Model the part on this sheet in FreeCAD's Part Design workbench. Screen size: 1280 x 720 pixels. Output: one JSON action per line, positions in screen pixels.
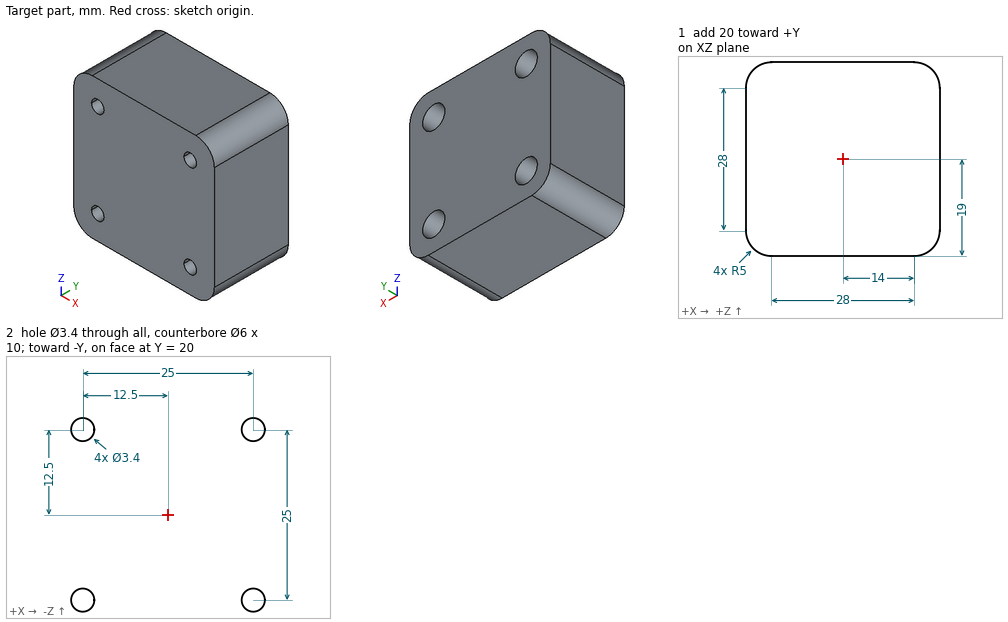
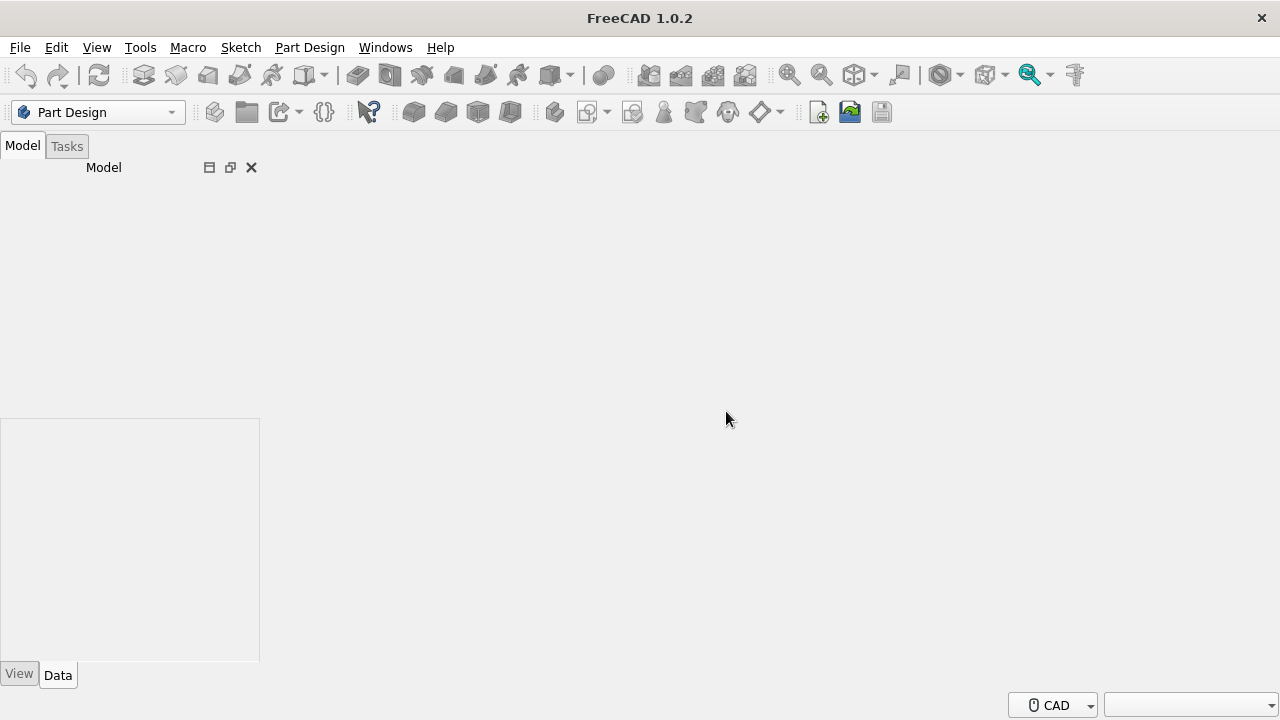
{"action": "left_click", "coordinate": [818, 112]}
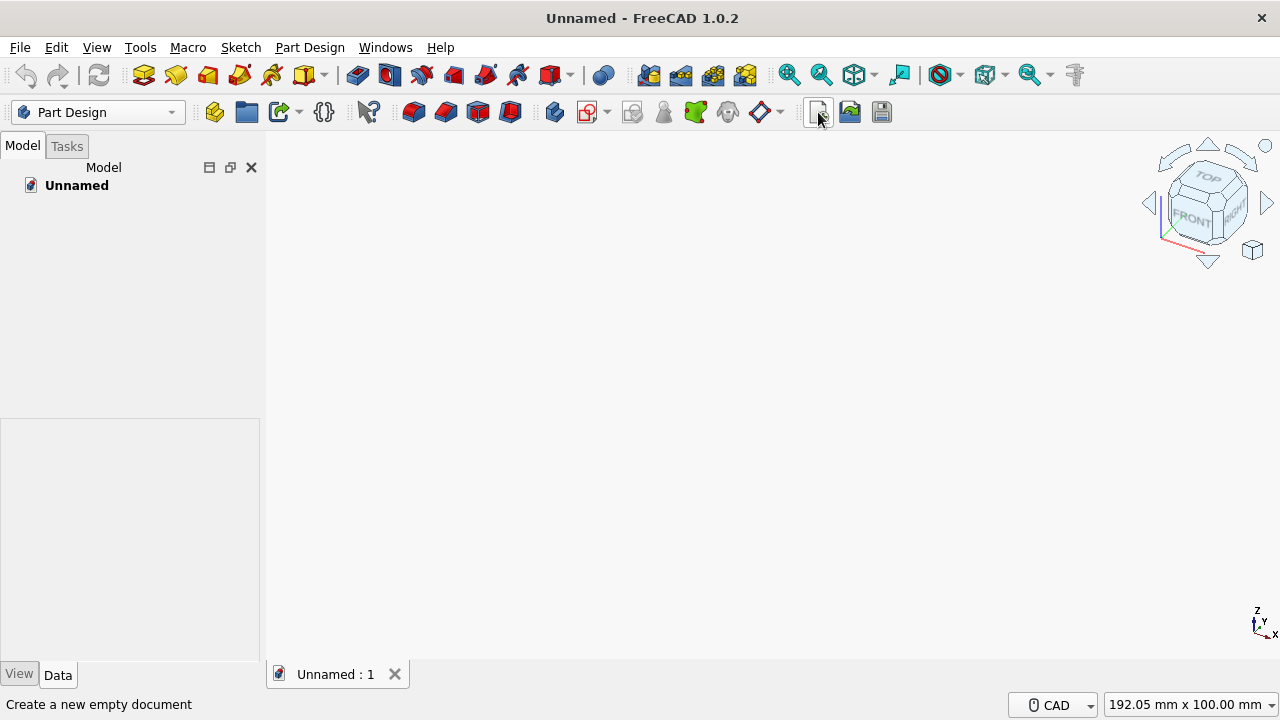
{"action": "left_click", "coordinate": [588, 112]}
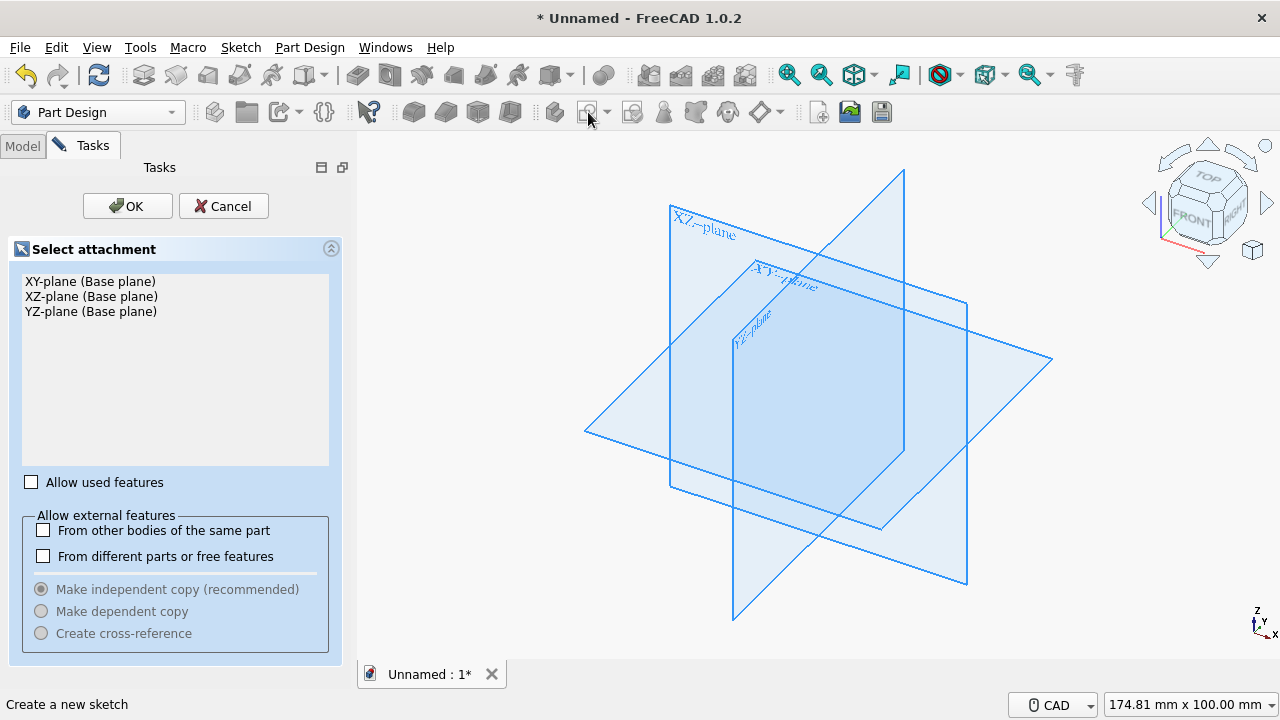
{"action": "left_click", "coordinate": [82, 296]}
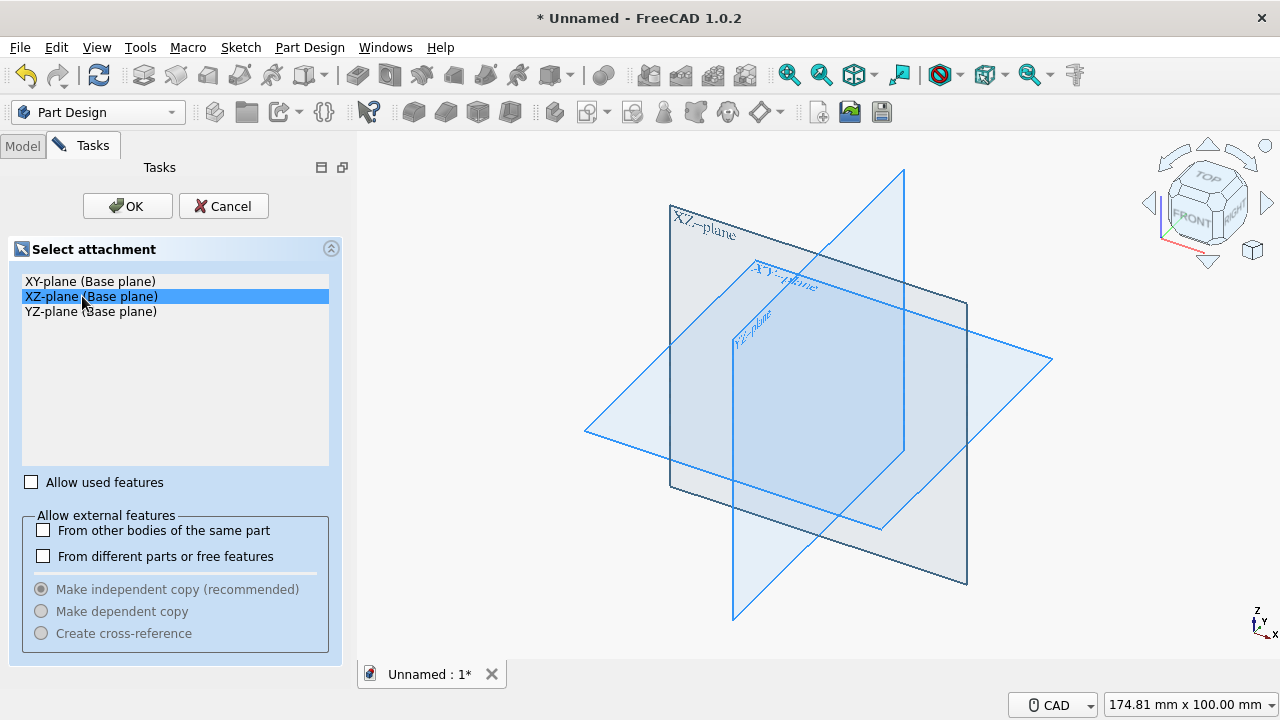
{"action": "left_click", "coordinate": [128, 206]}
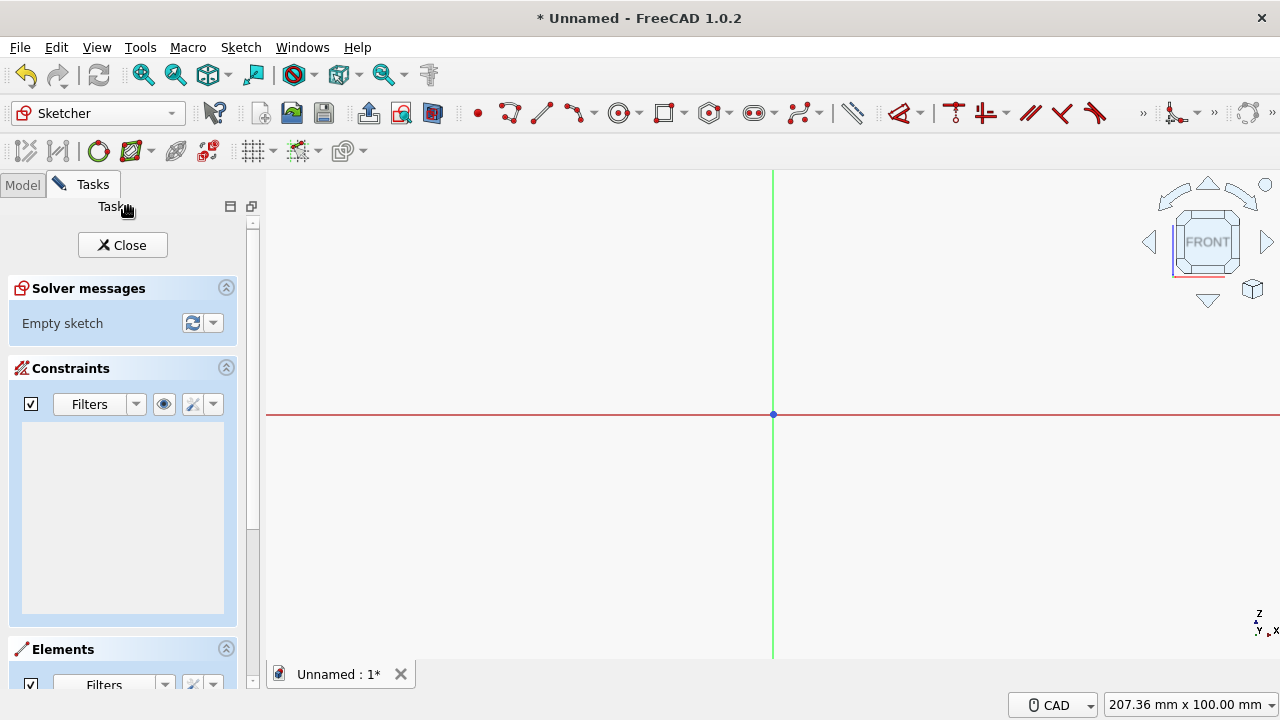
{"action": "scroll", "coordinate": [912, 414], "scroll_direction": "up", "scroll_amount": 2}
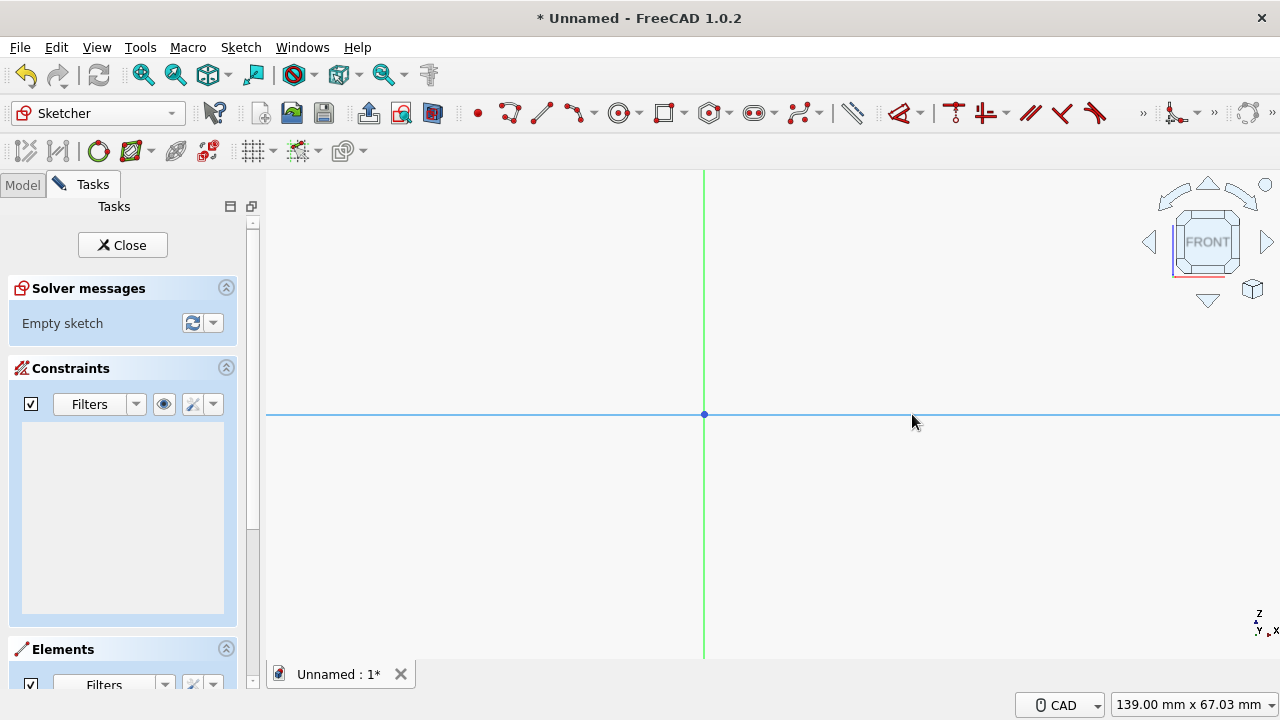
{"action": "left_click", "coordinate": [542, 114]}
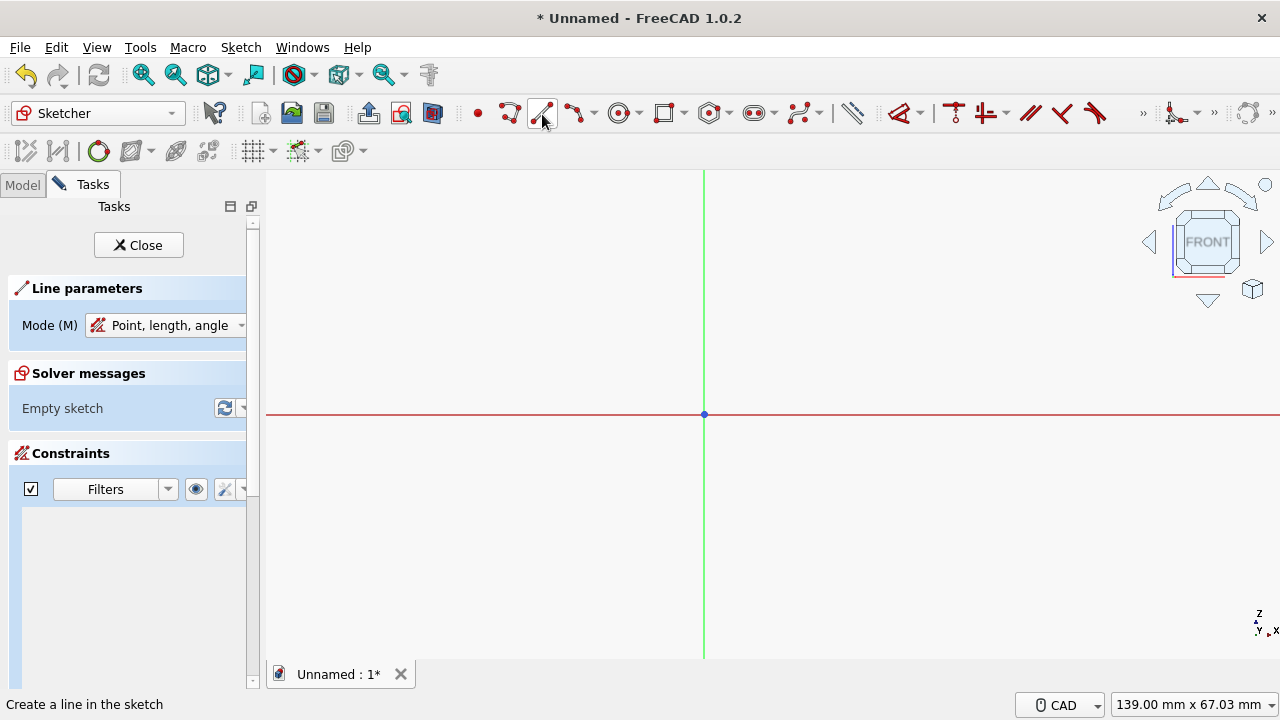
{"action": "left_click", "coordinate": [806, 553]}
{"action": "left_click", "coordinate": [602, 553]}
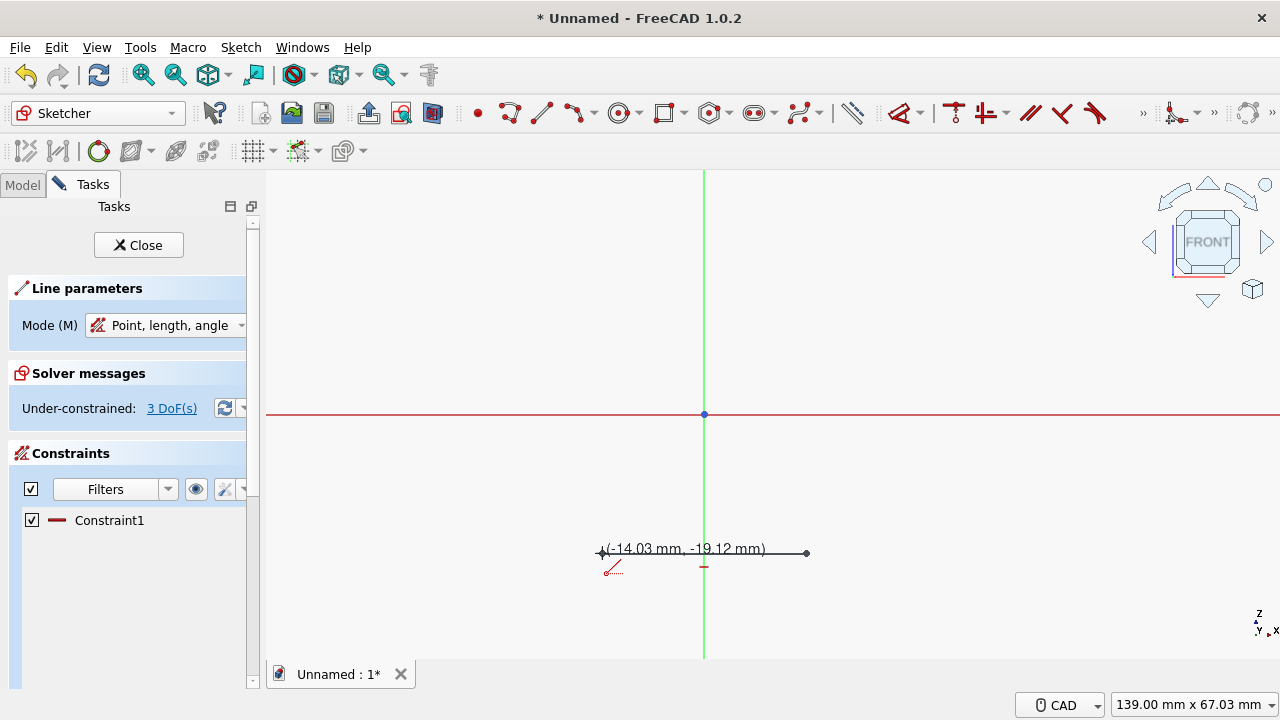
{"action": "left_click", "coordinate": [566, 517]}
{"action": "left_click", "coordinate": [566, 312]}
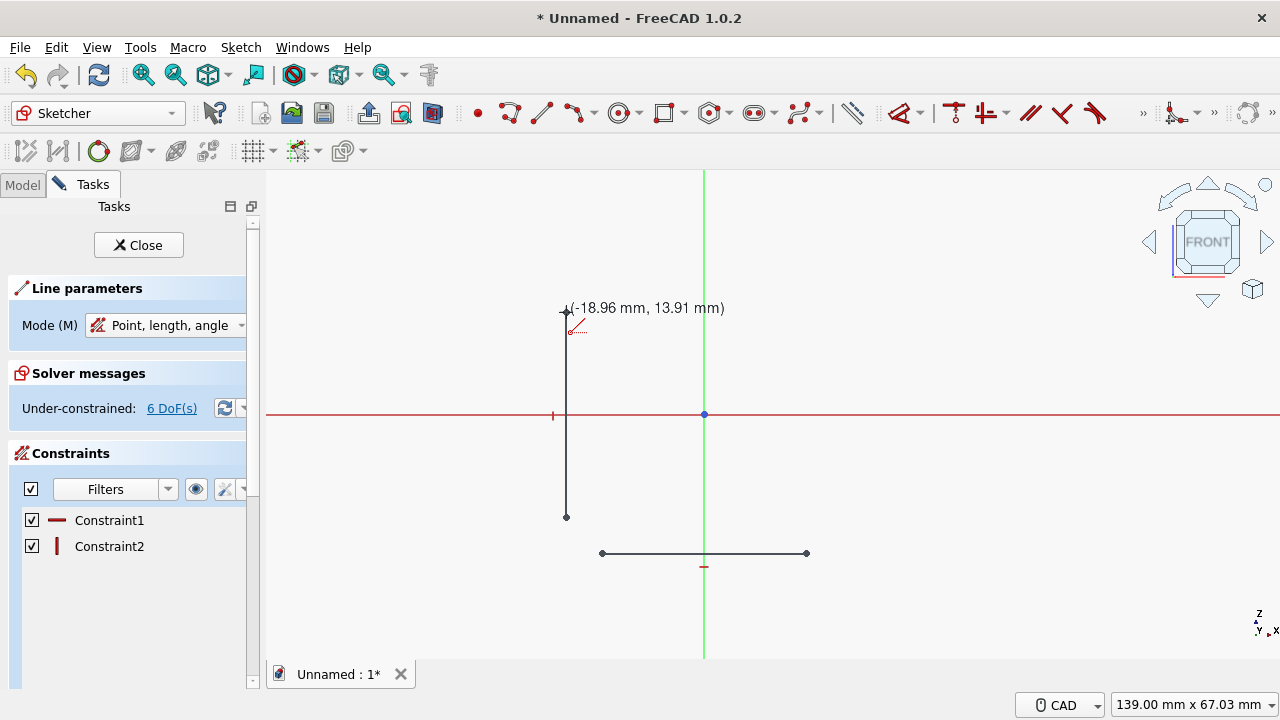
{"action": "left_click", "coordinate": [602, 276]}
{"action": "left_click", "coordinate": [806, 276]}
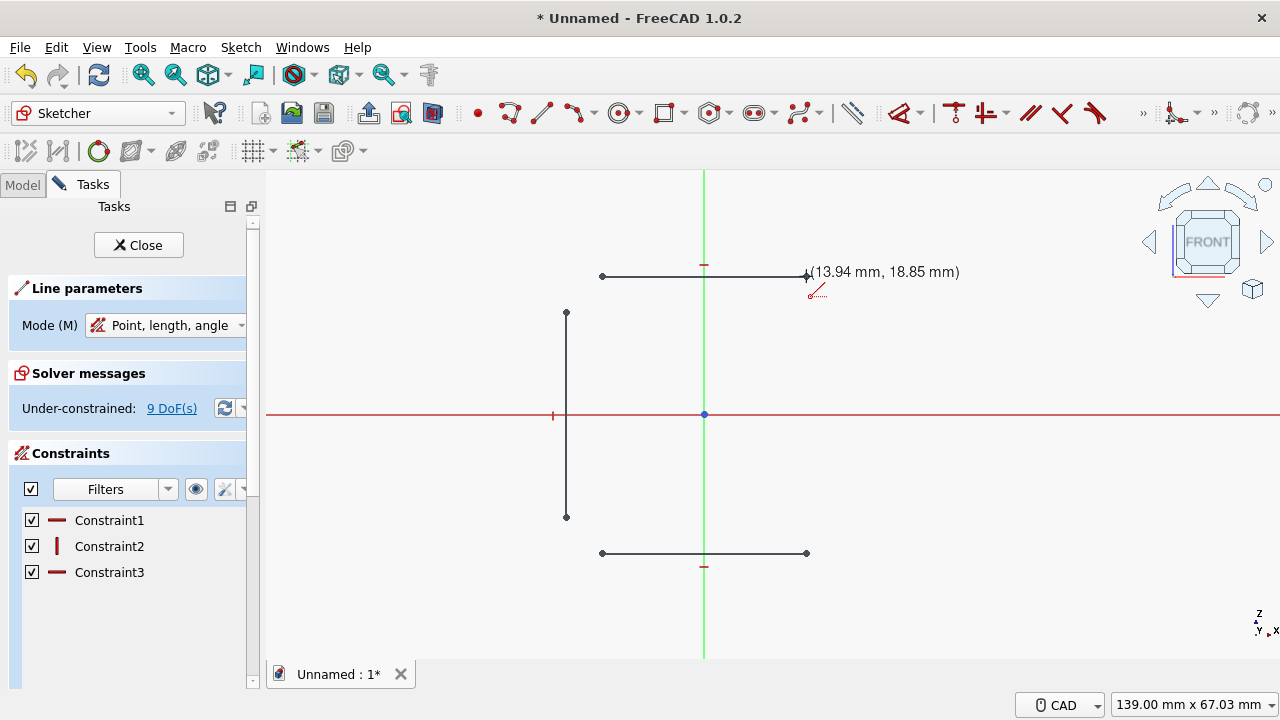
{"action": "left_click", "coordinate": [843, 312]}
{"action": "left_click", "coordinate": [843, 517]}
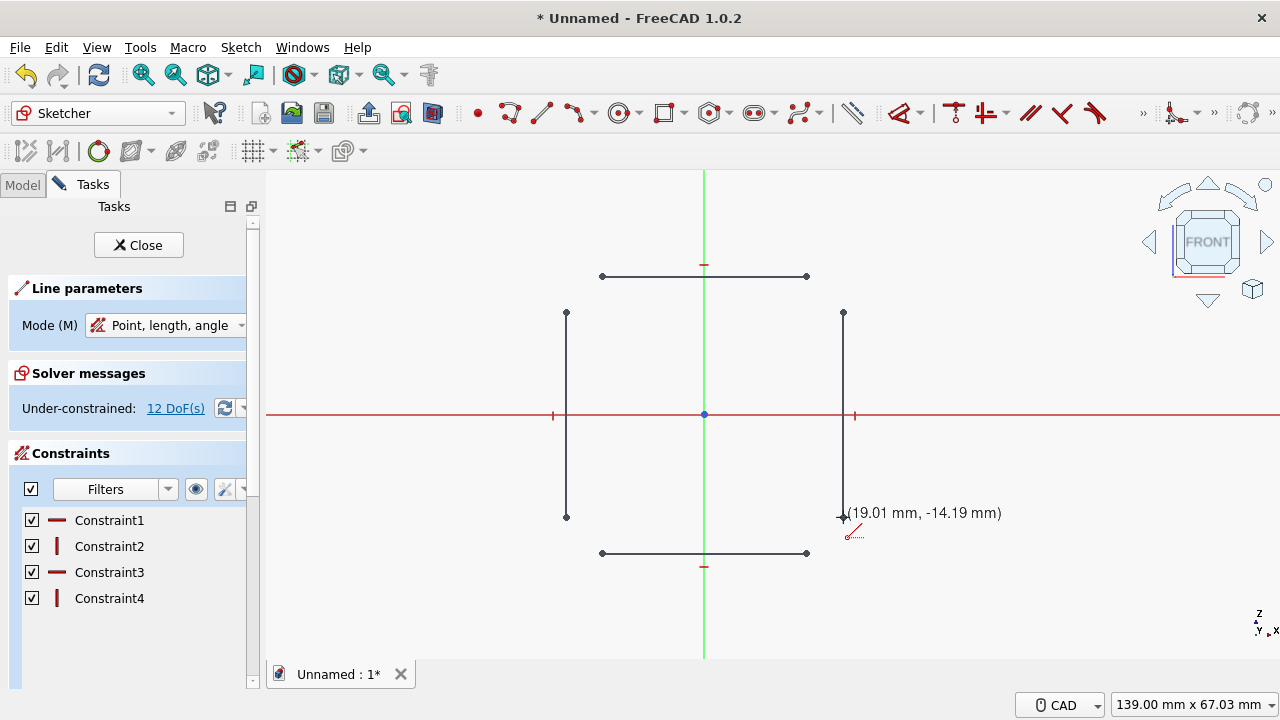
{"action": "left_click", "coordinate": [574, 114]}